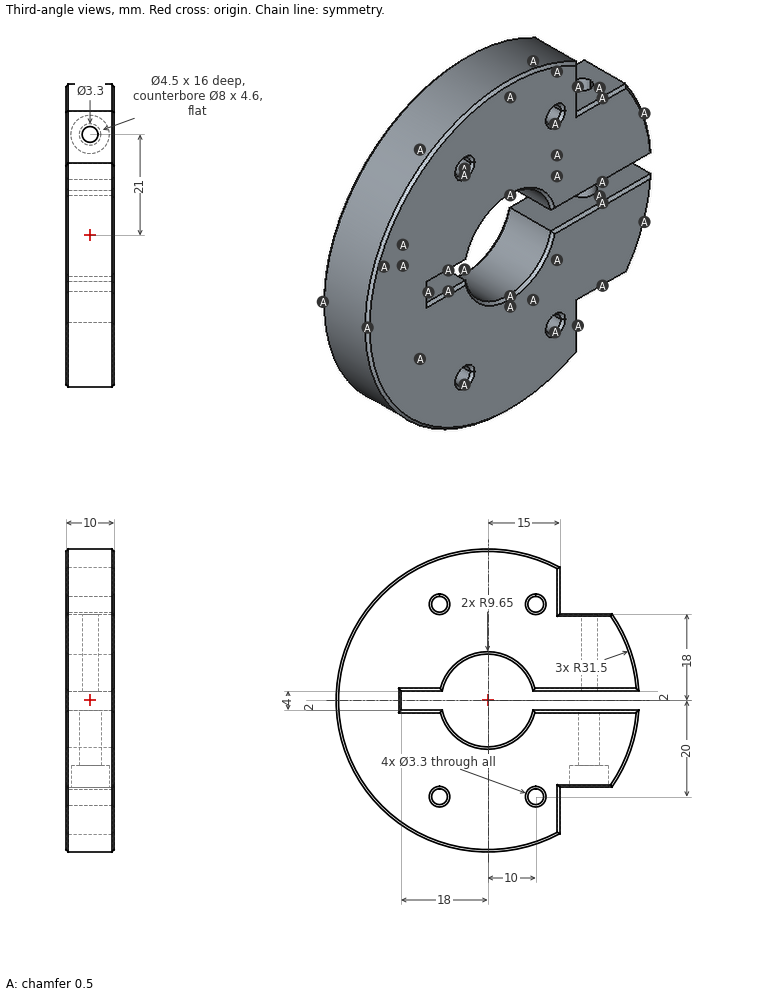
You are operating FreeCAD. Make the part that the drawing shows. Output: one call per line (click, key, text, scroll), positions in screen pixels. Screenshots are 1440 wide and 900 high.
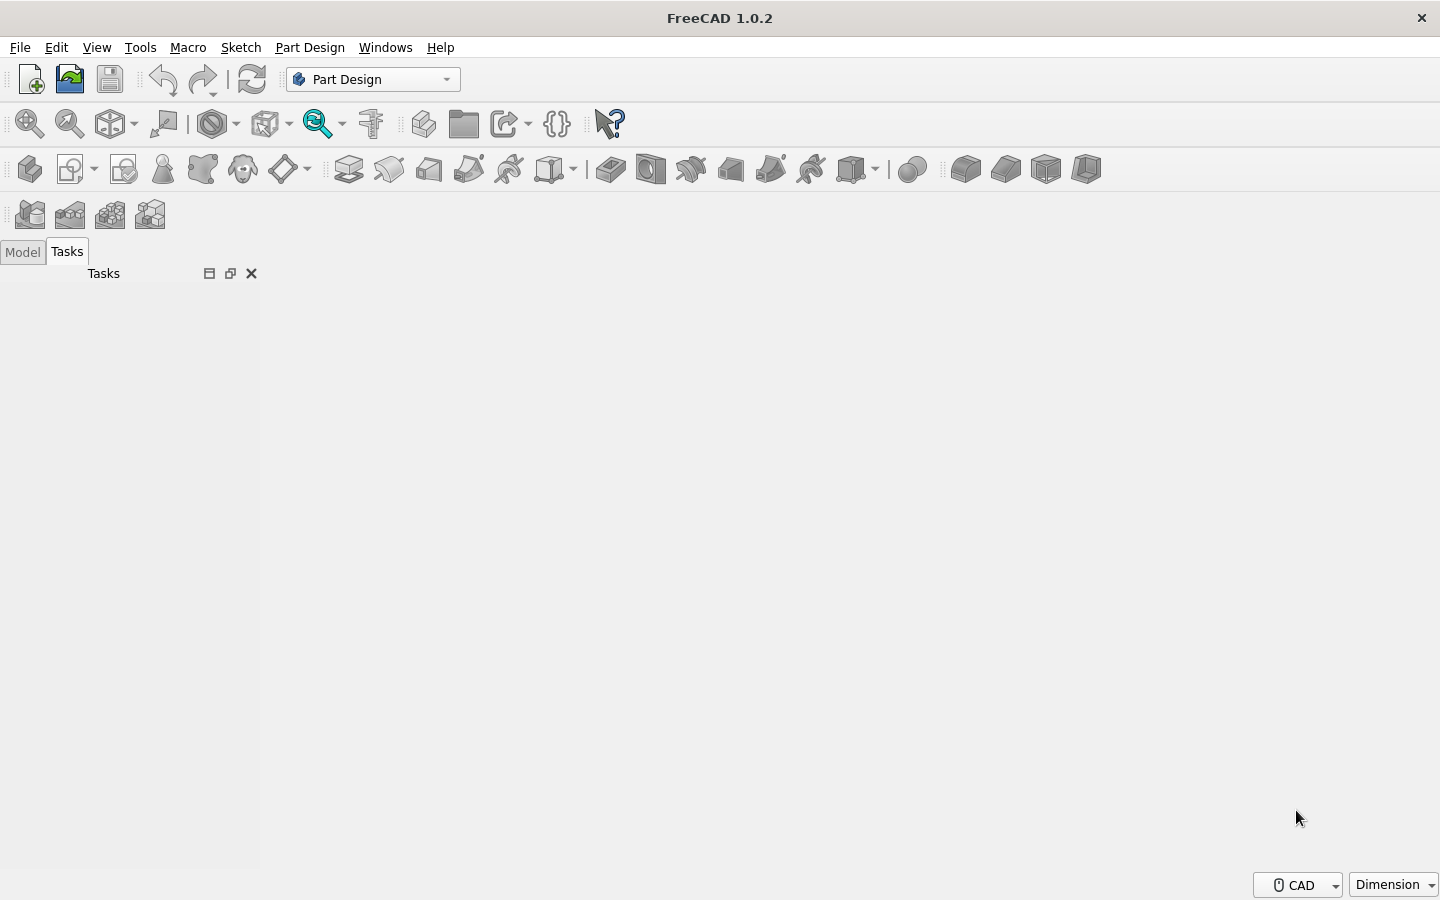
click(30, 80)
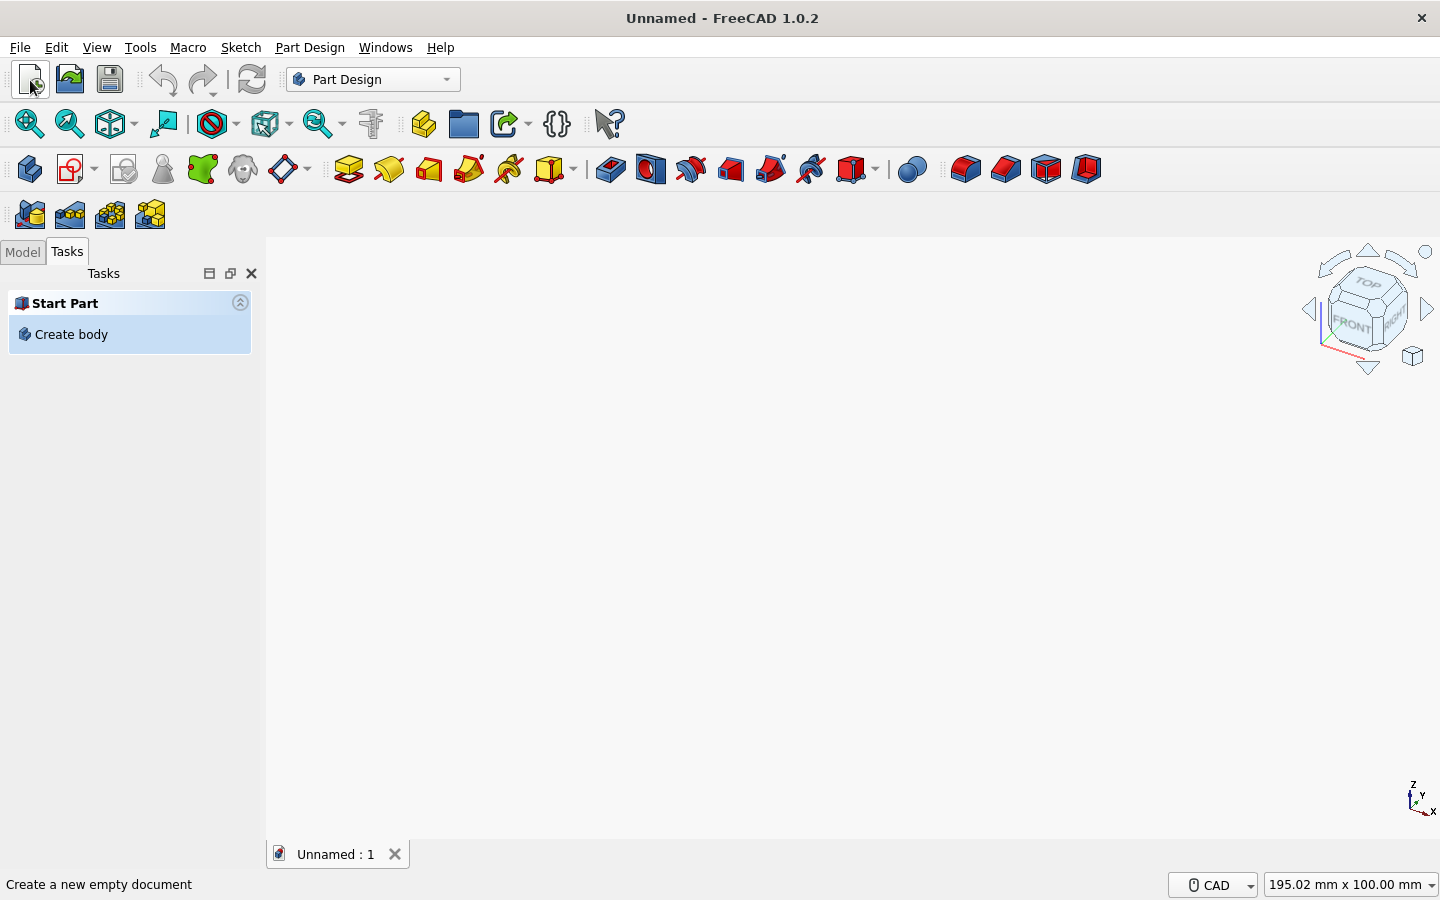
click(70, 170)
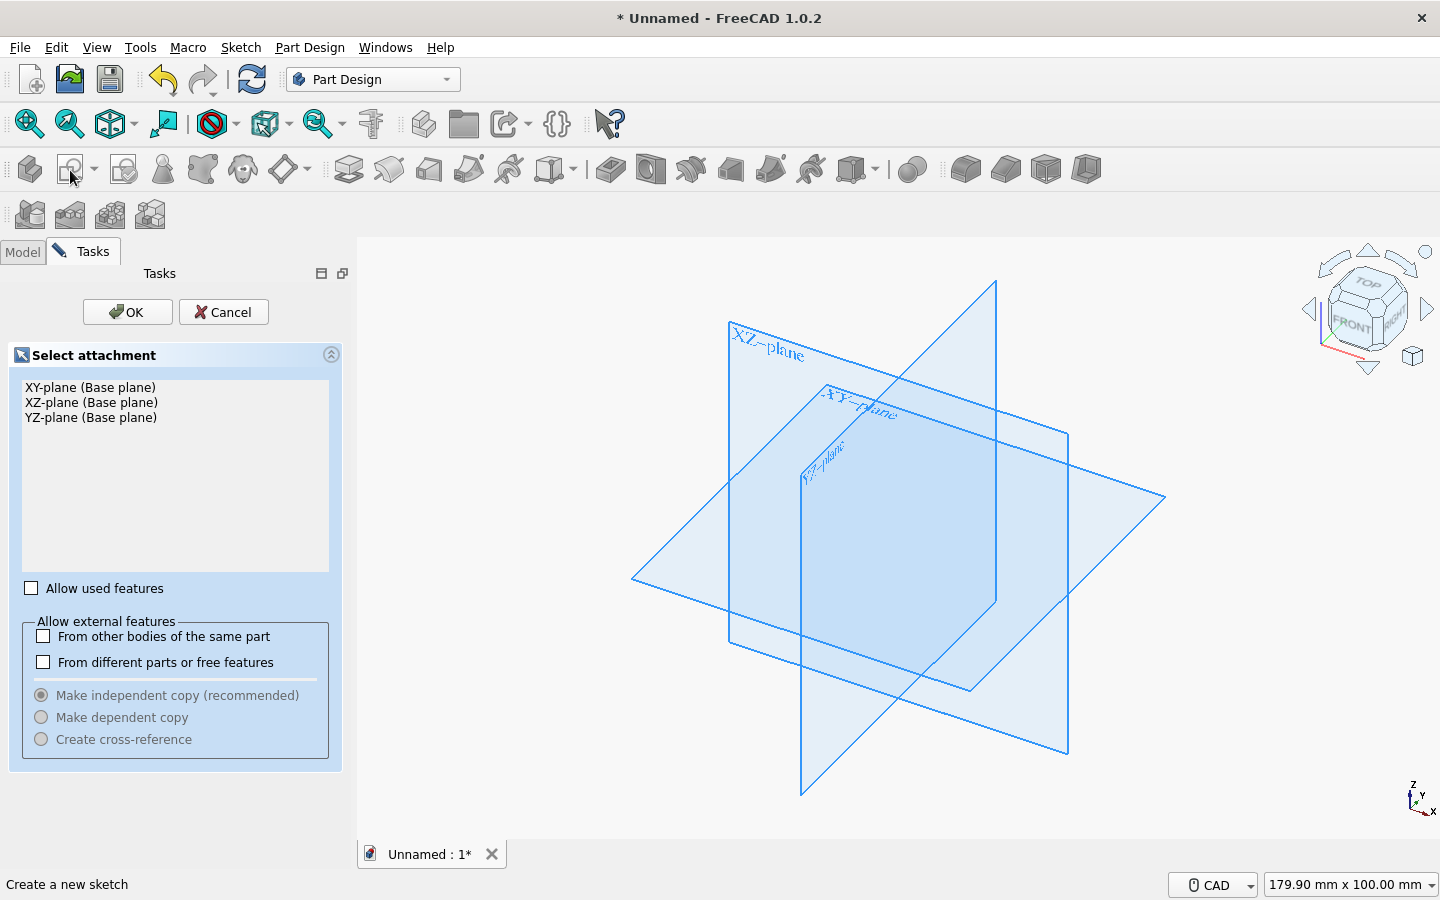
click(82, 418)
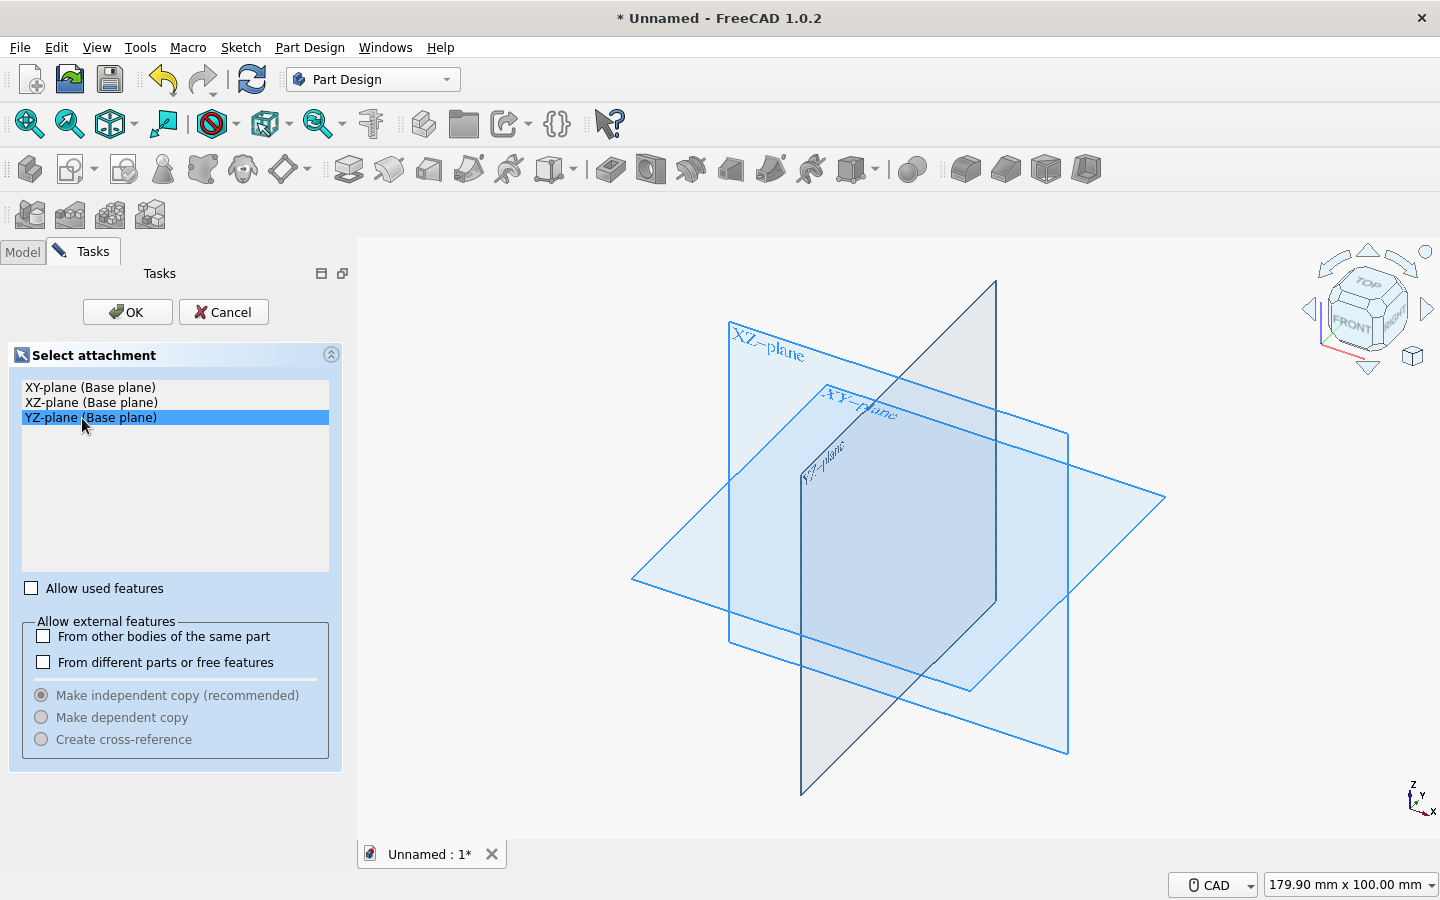
click(128, 312)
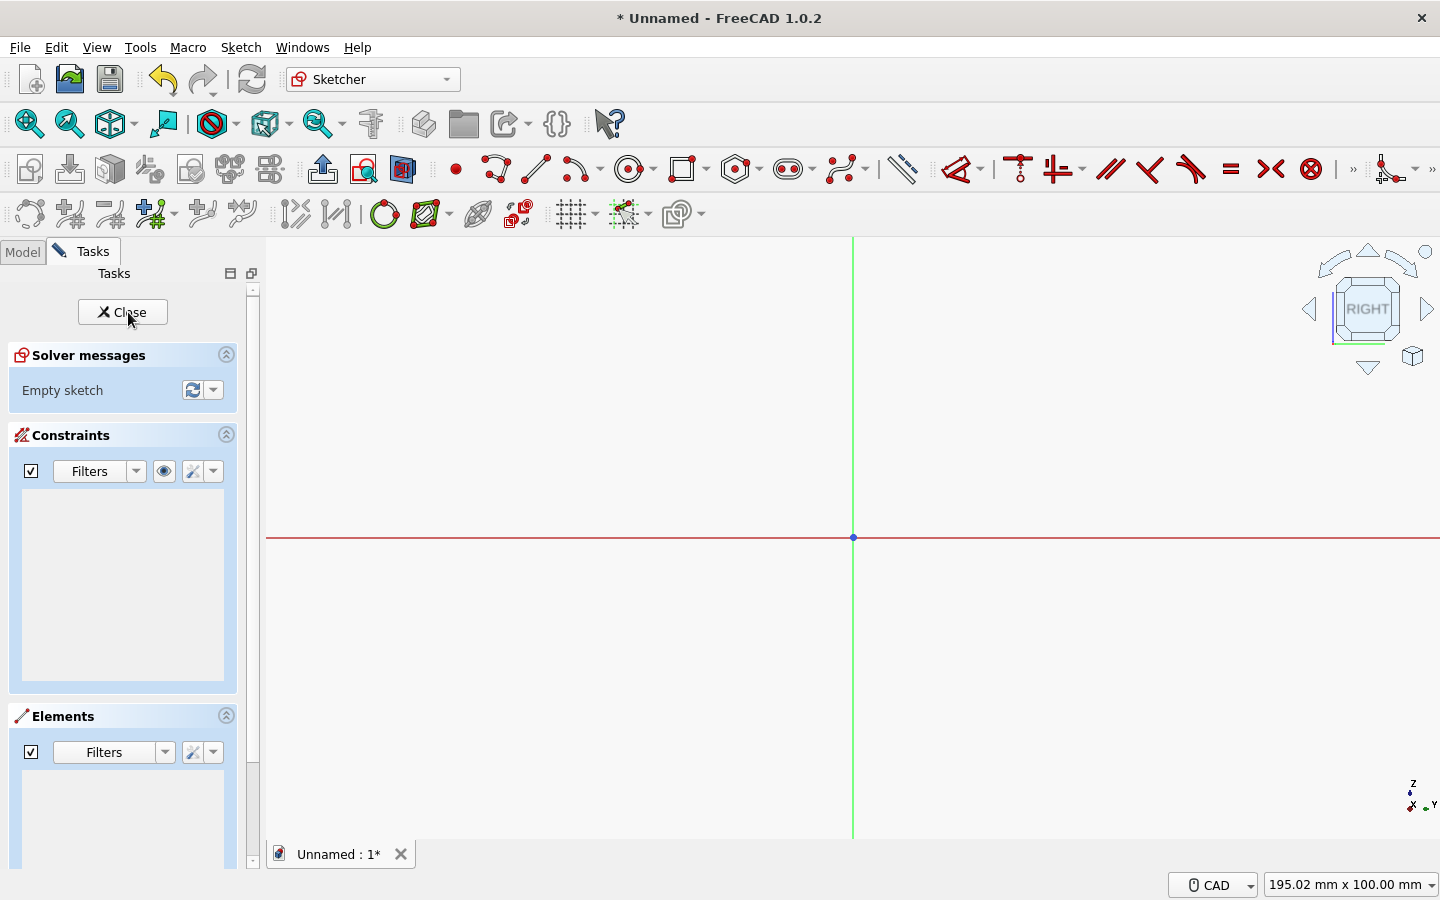
key(g)
key(m)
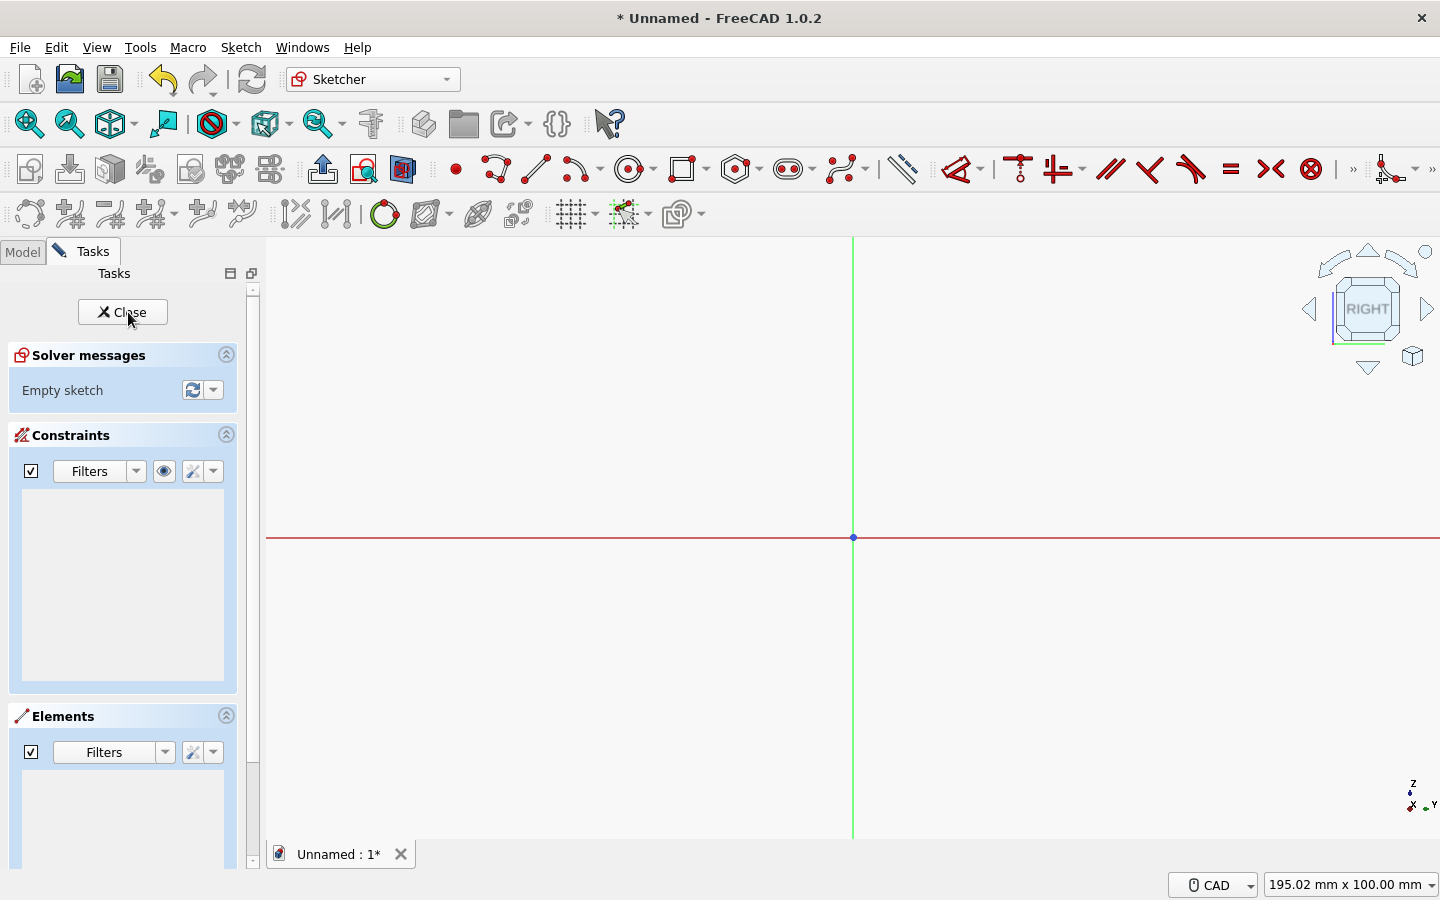
scroll(796, 550, up, 2)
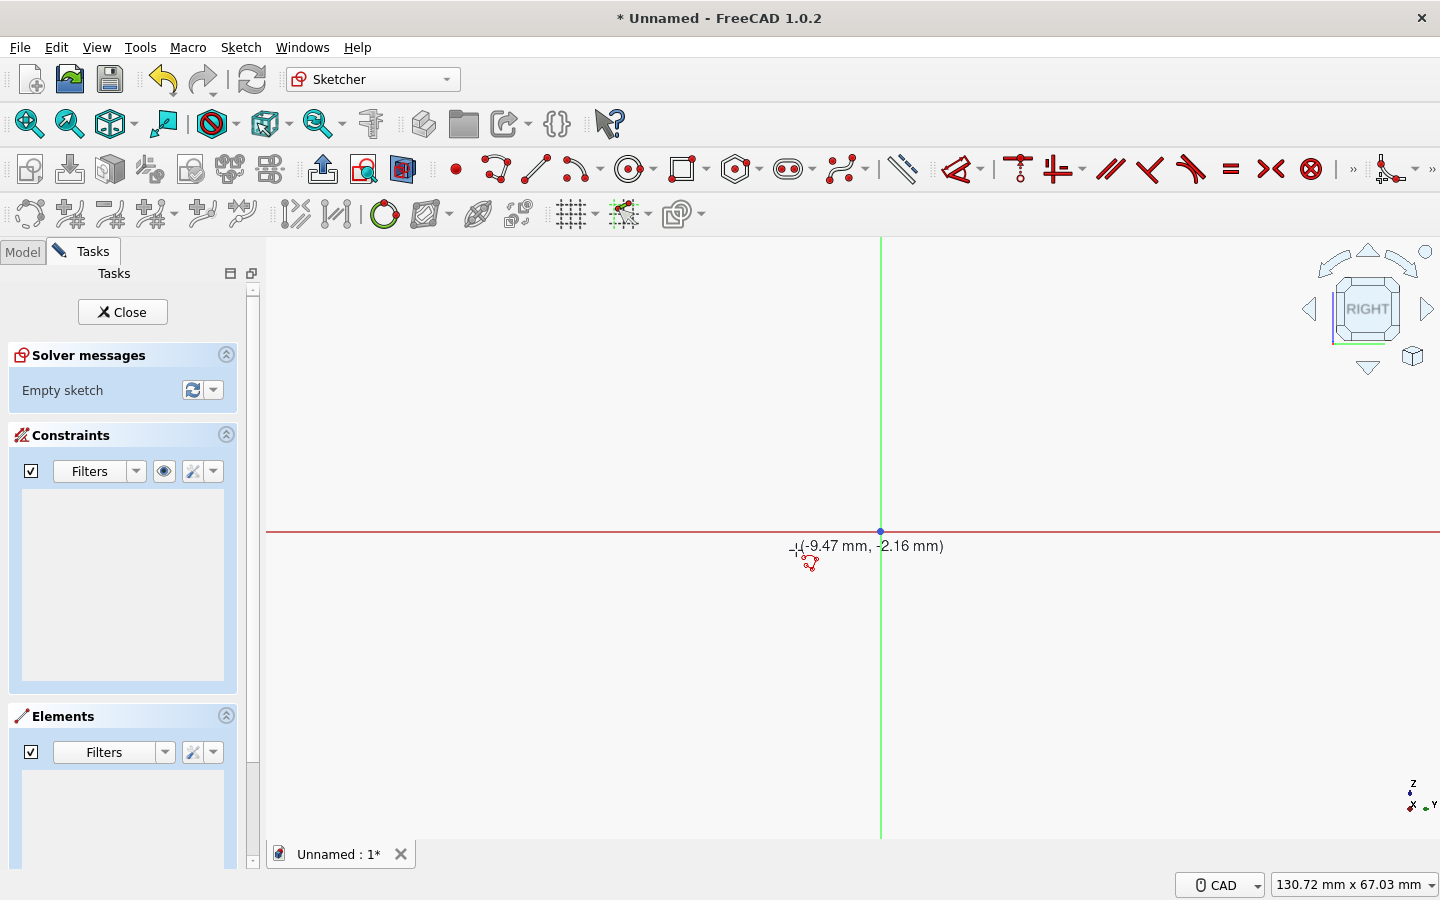
click(796, 550)
click(719, 550)
click(719, 514)
click(796, 514)
right_click(796, 514)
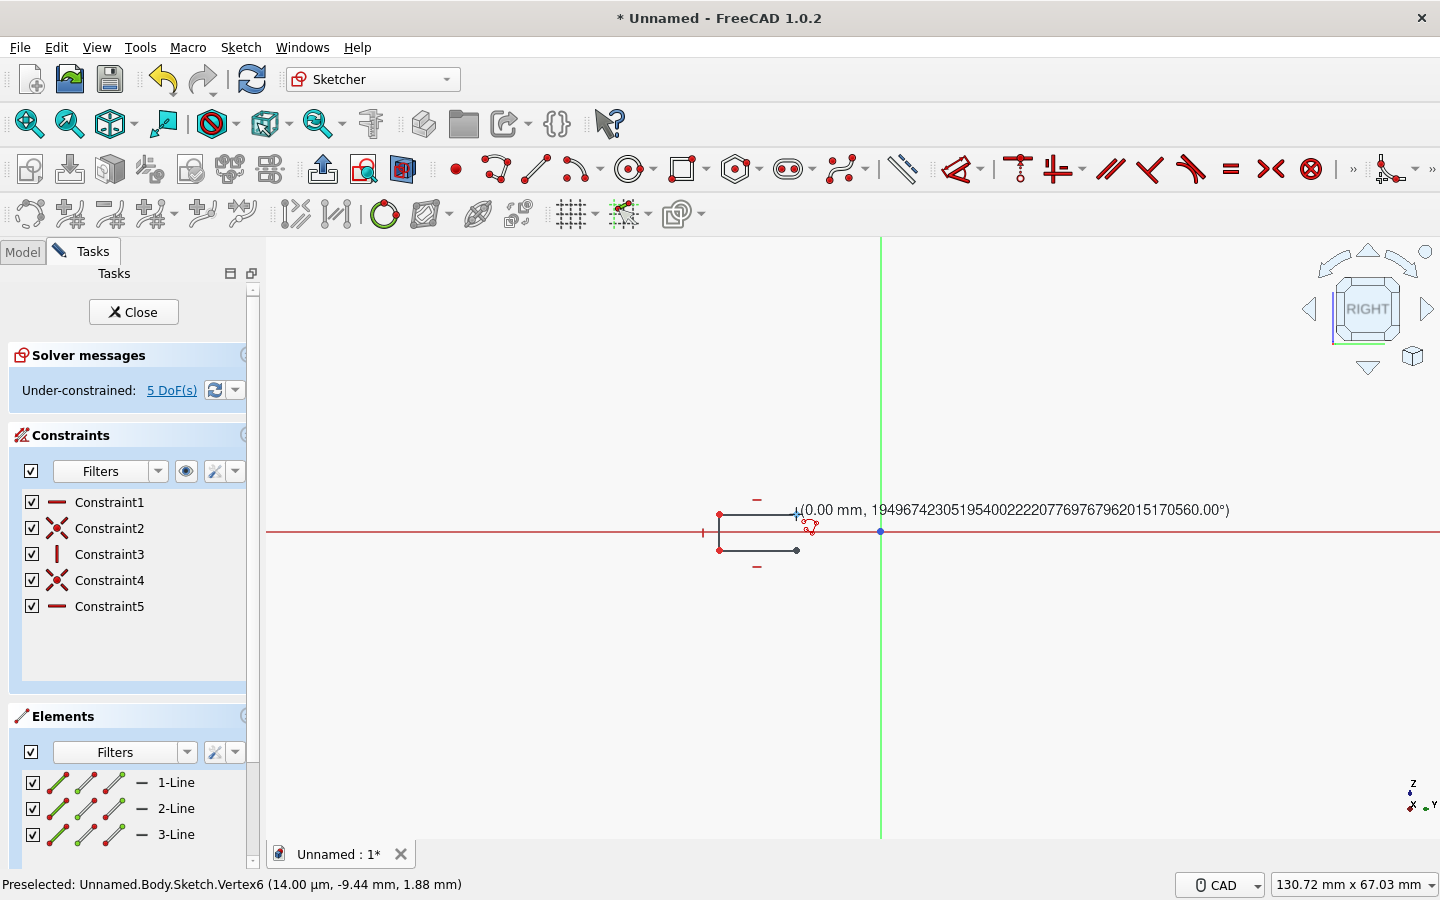
key(g)
key(l)